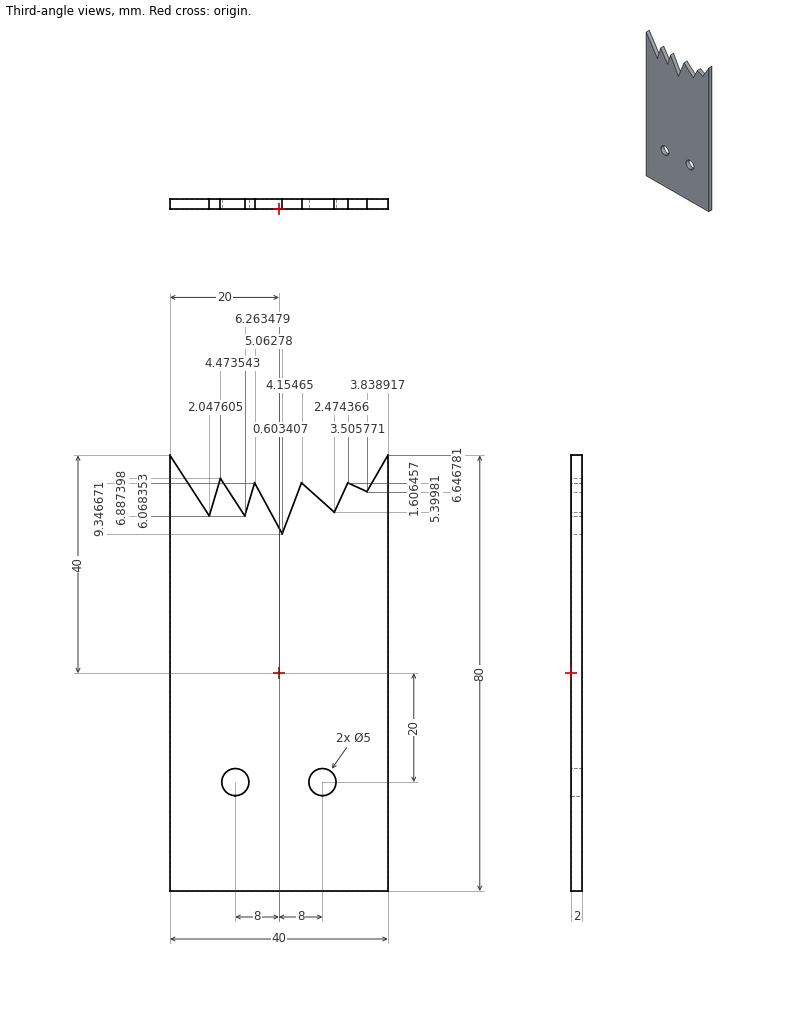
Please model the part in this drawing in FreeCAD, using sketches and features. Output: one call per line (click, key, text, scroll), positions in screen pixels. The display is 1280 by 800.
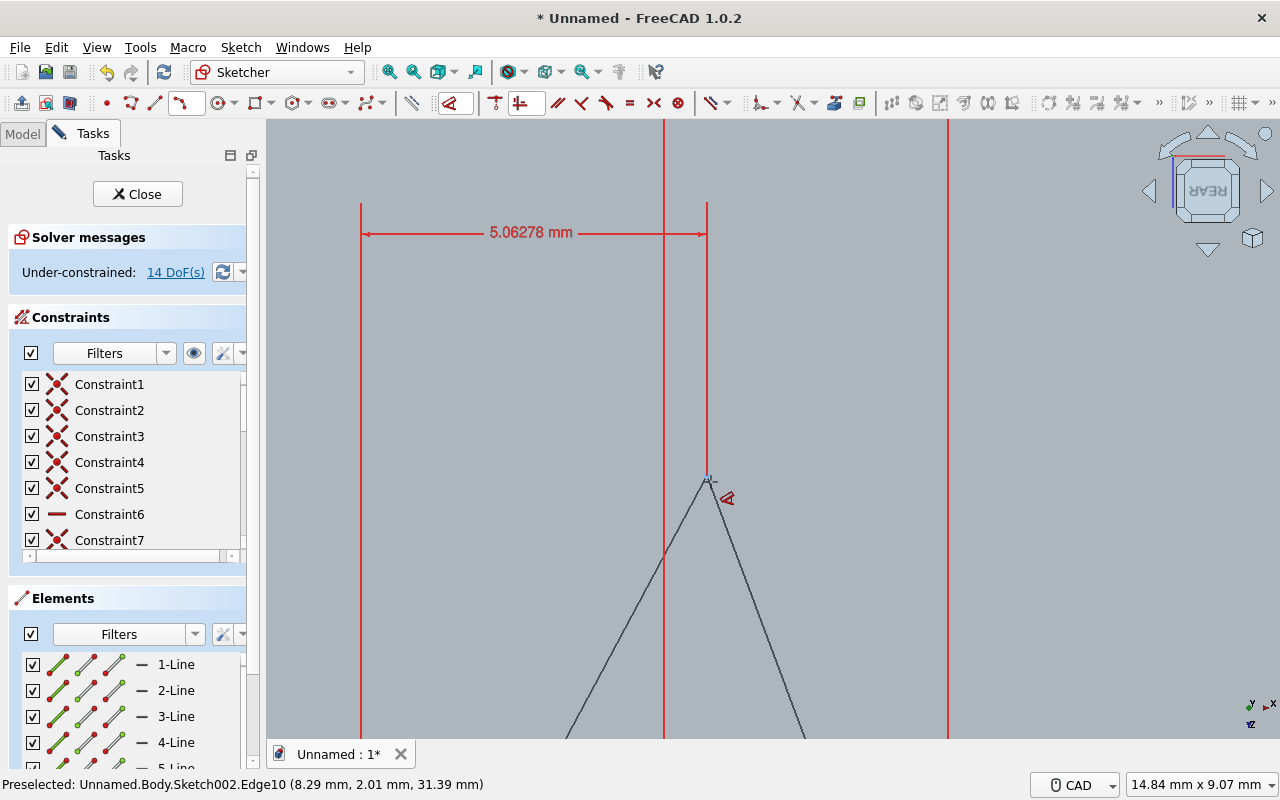
click(707, 476)
click(695, 534)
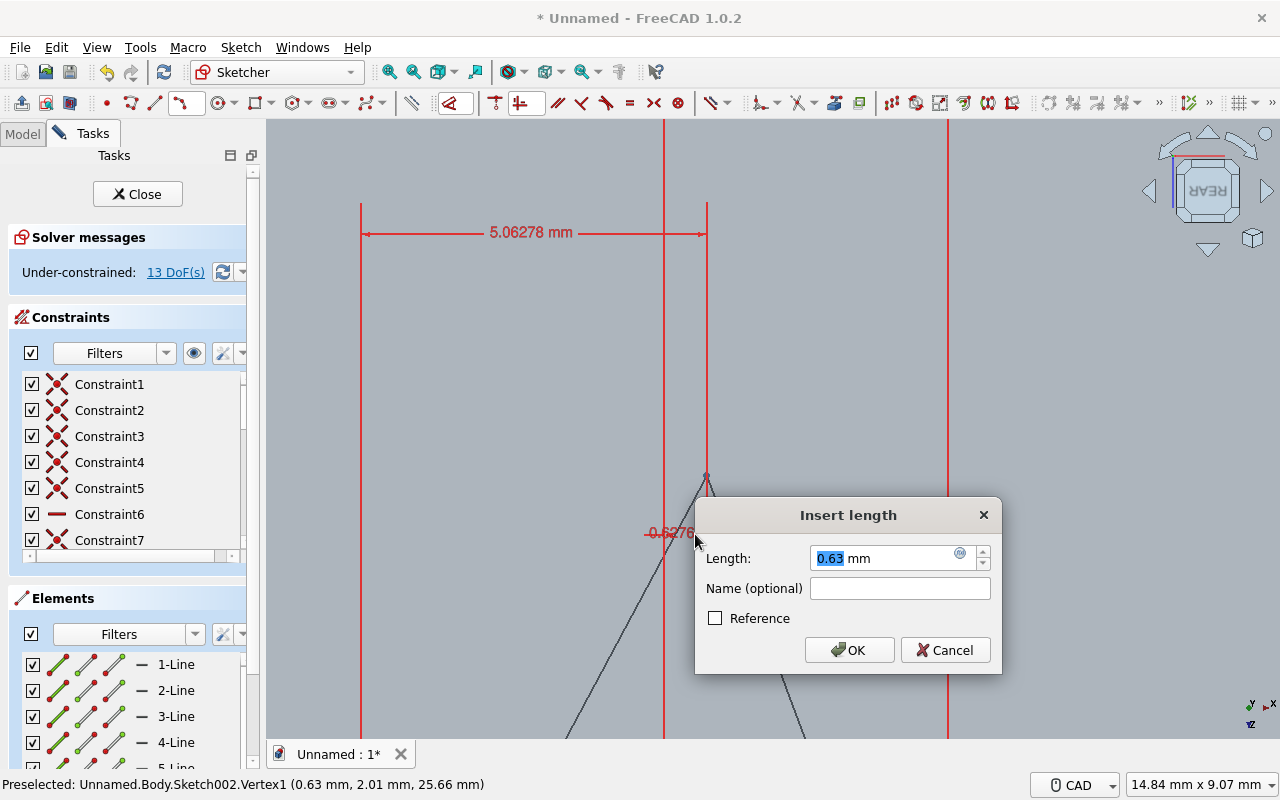
text(0.603407)
key(Return)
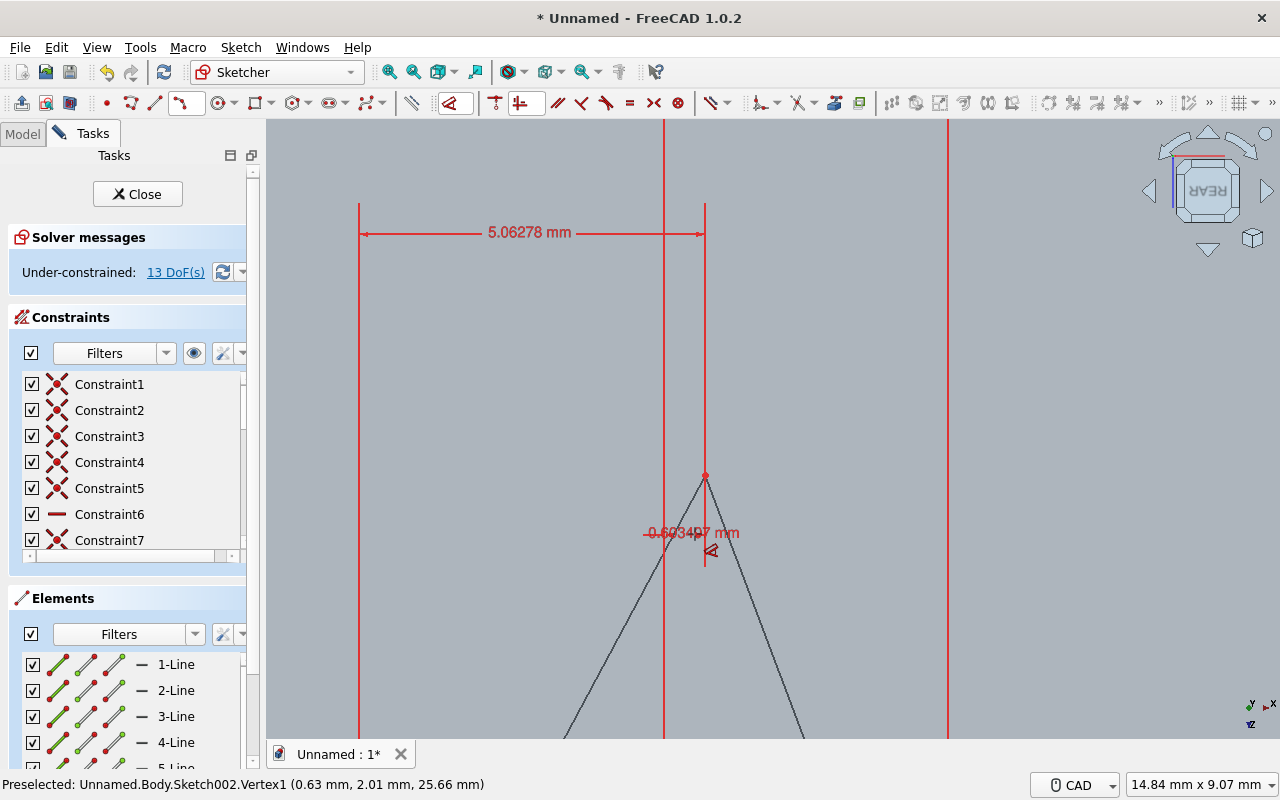
scroll(711, 482, down, 10)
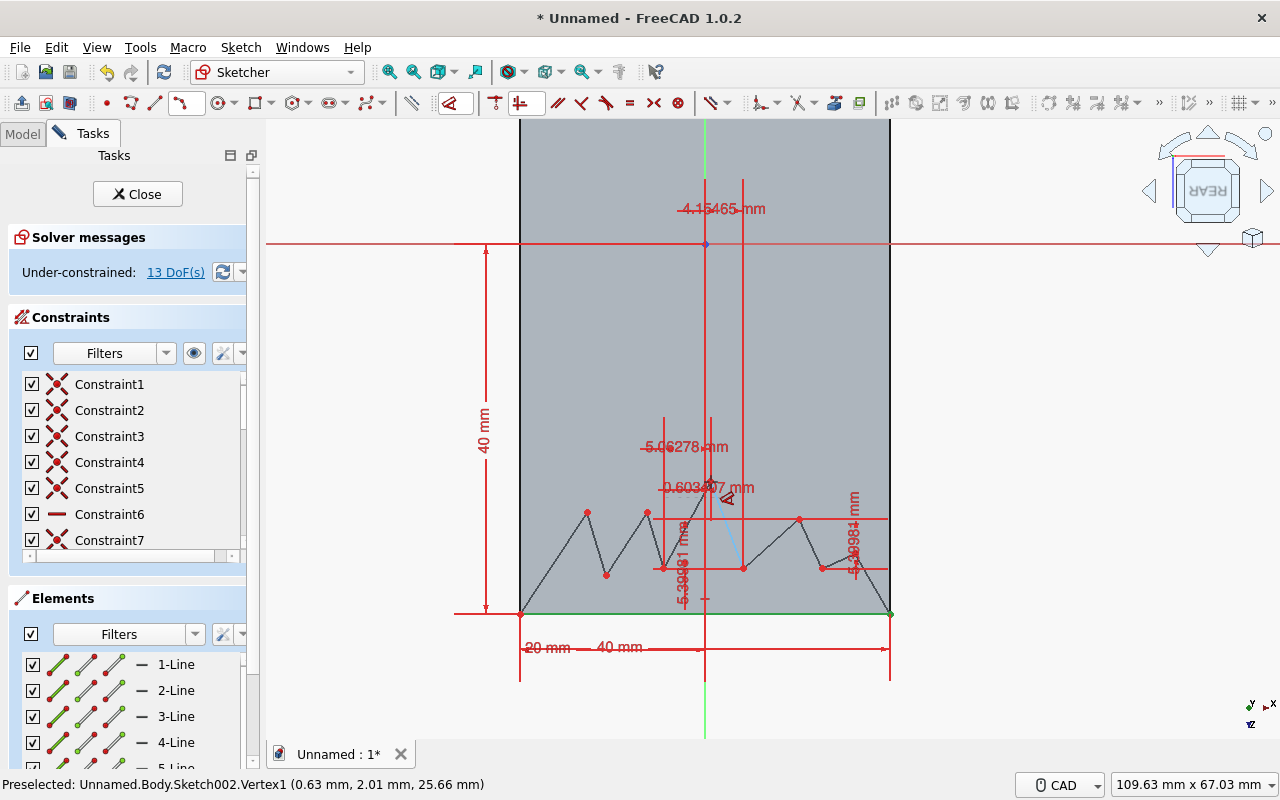
click(647, 513)
click(676, 186)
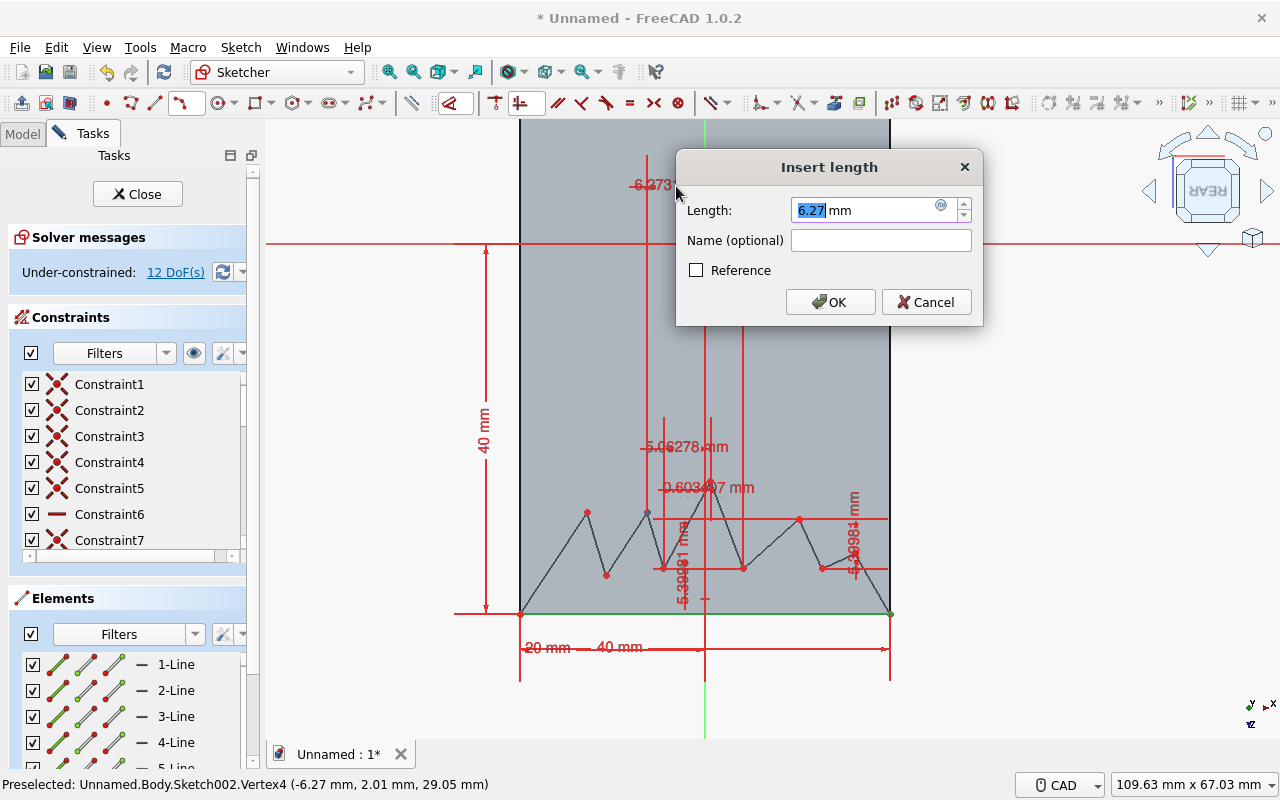
text(6.263479)
key(Return)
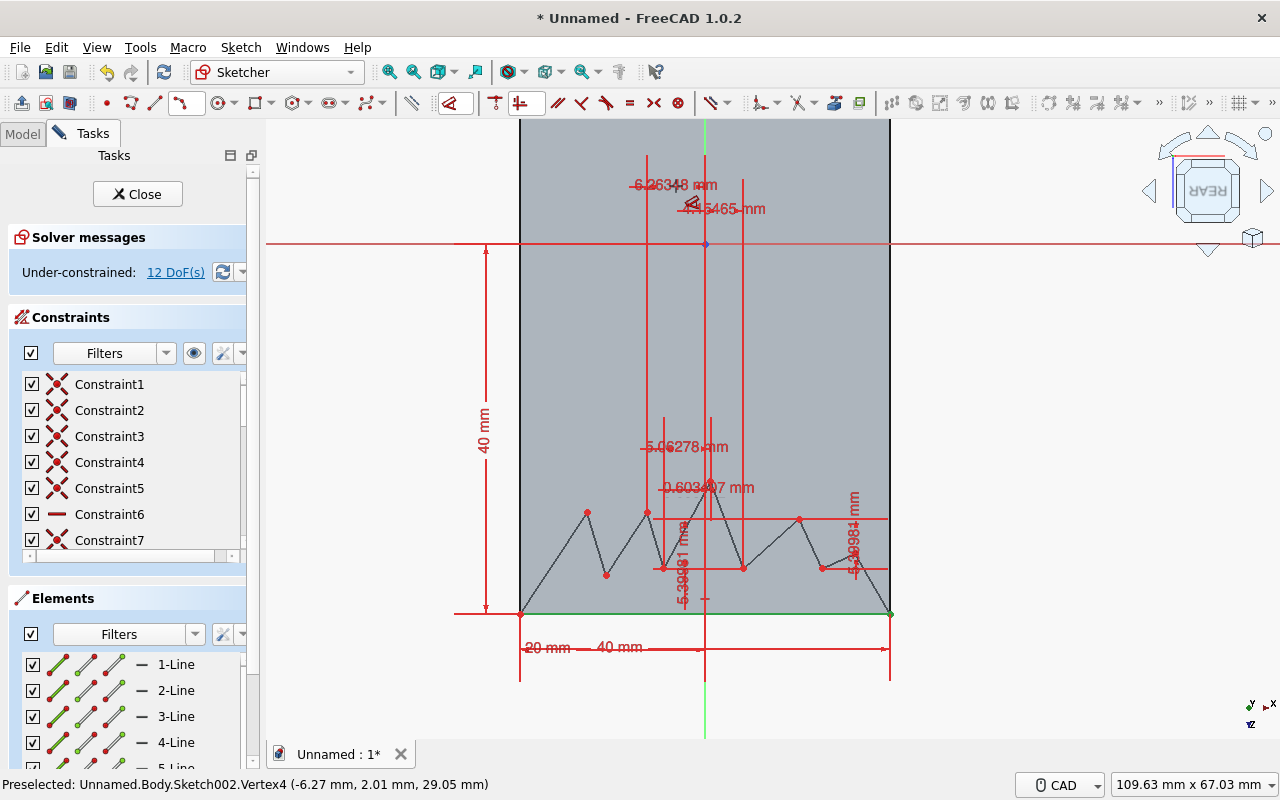
click(678, 543)
click(630, 505)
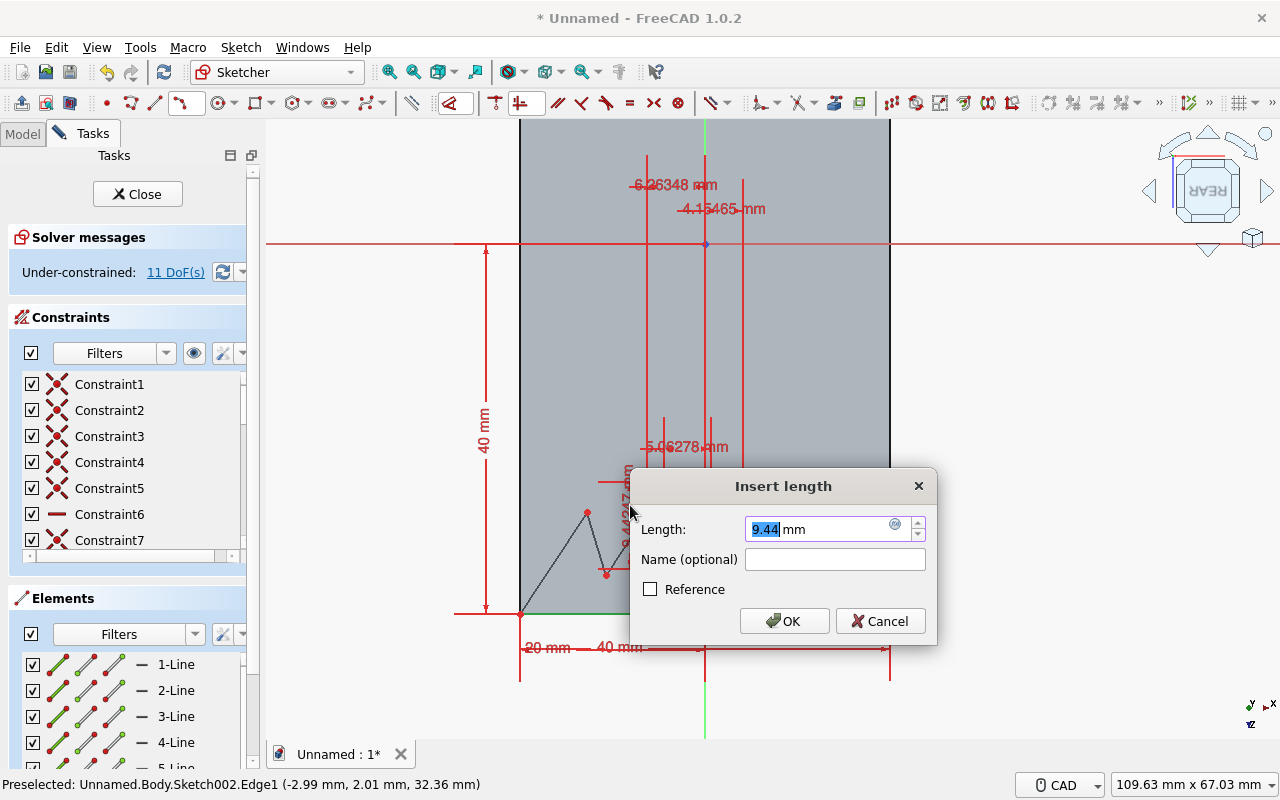
text(9.346671)
key(Return)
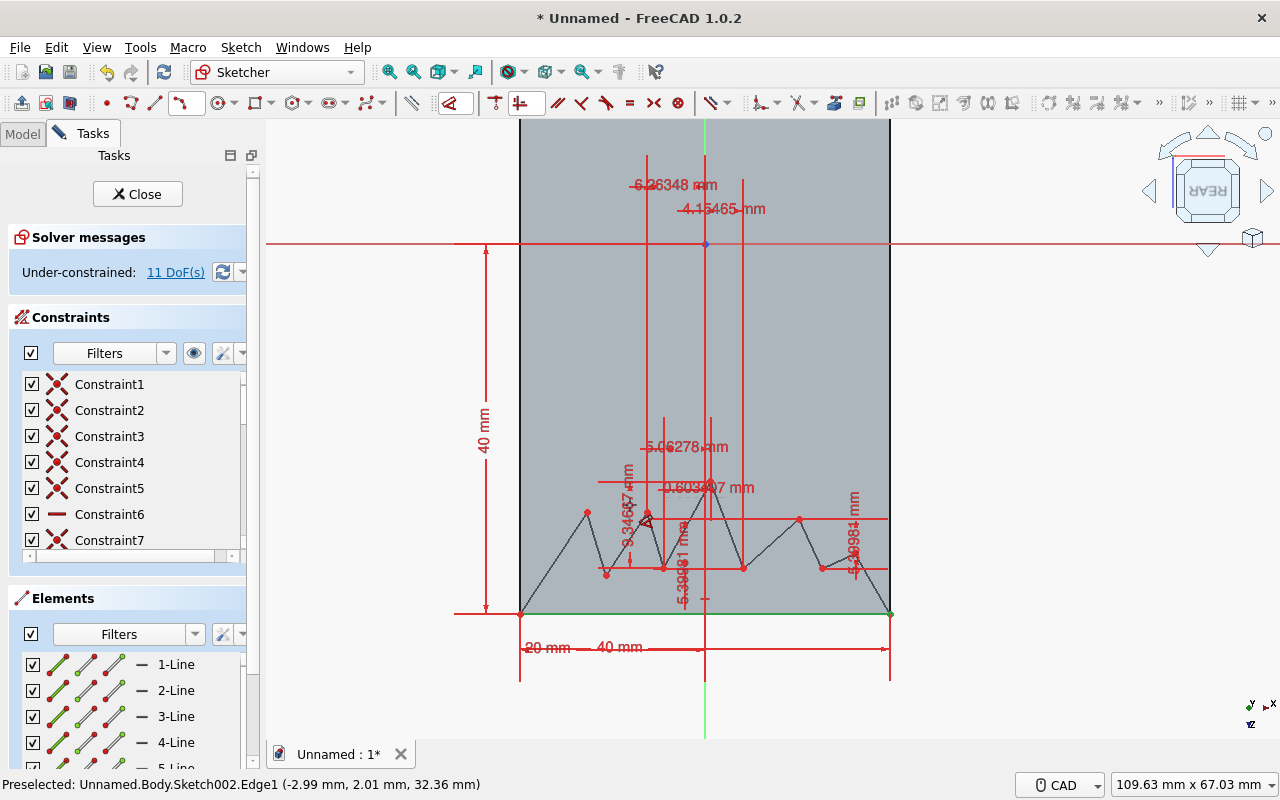
click(659, 552)
click(613, 541)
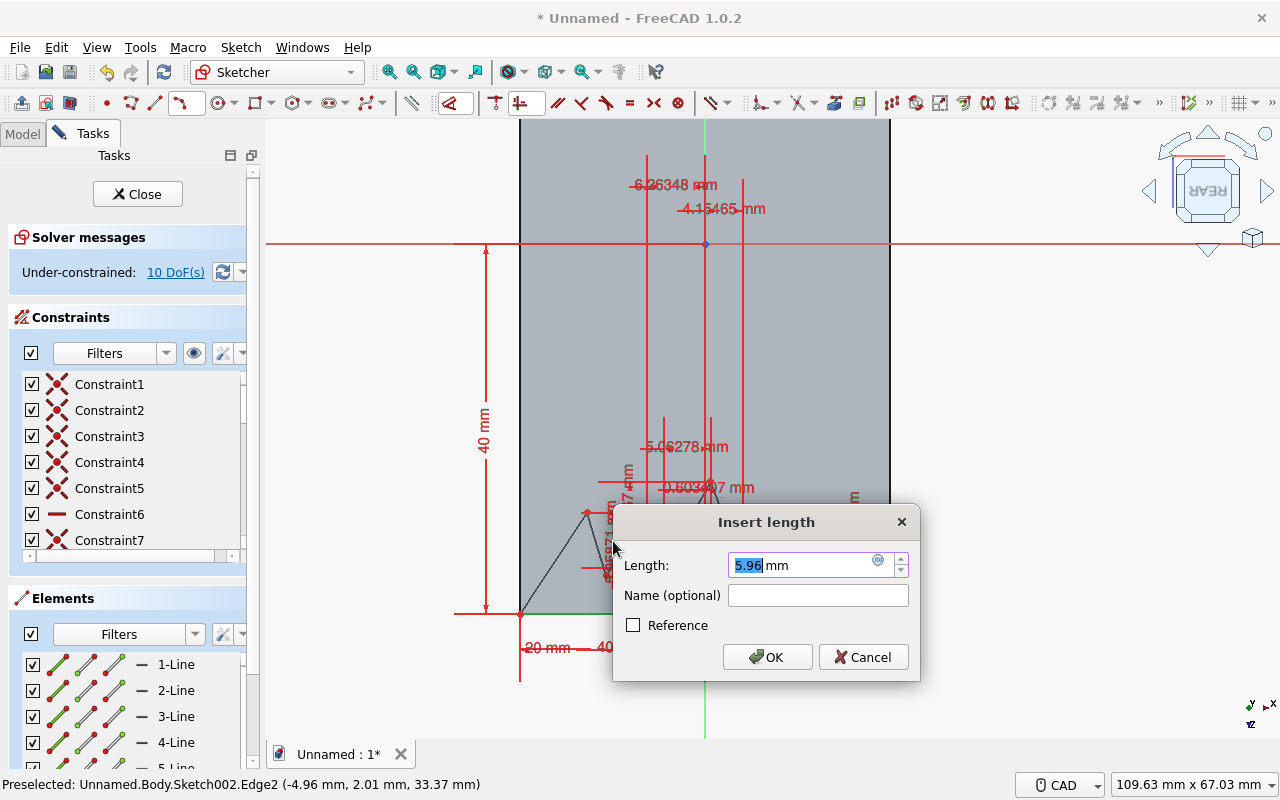
text(6.068353)
key(Return)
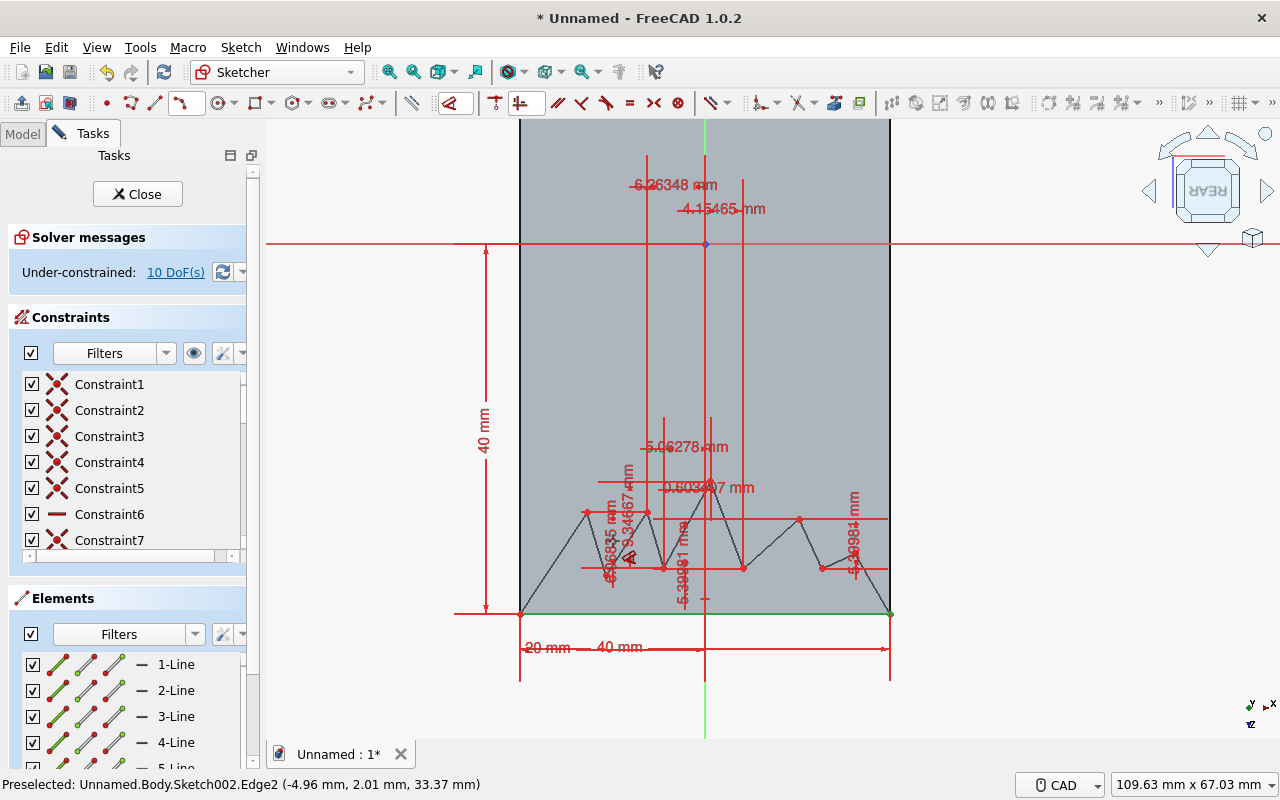
click(635, 531)
click(627, 478)